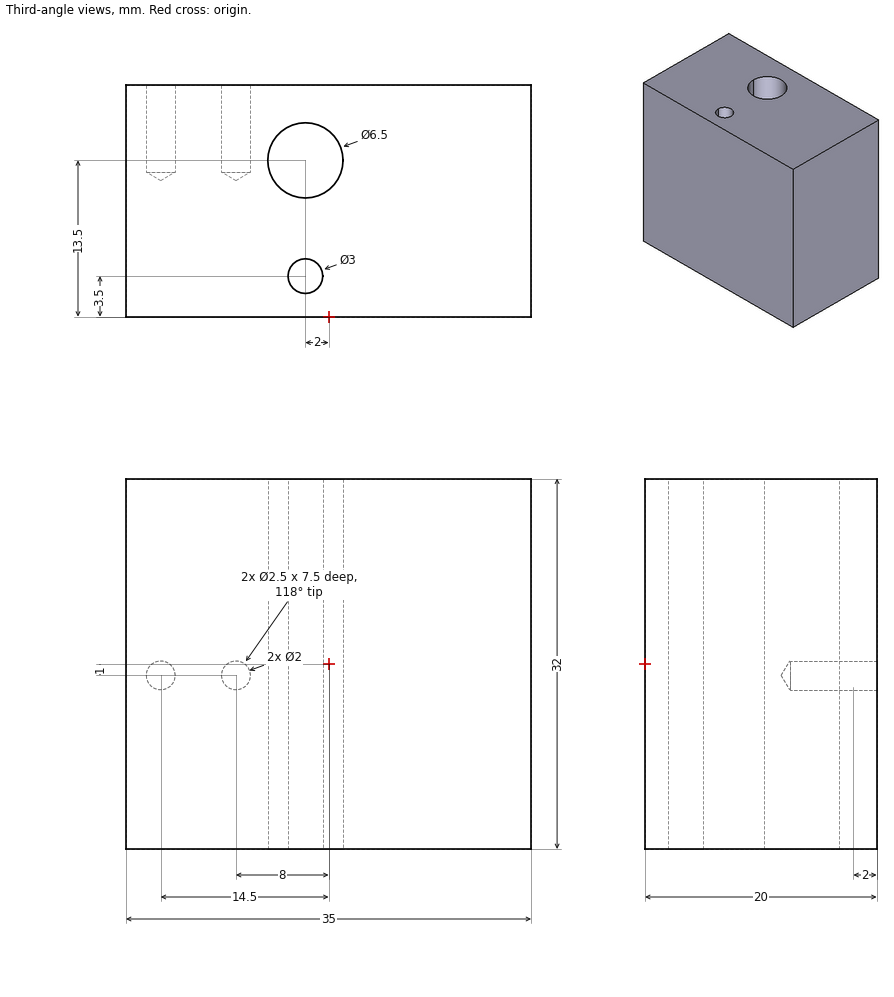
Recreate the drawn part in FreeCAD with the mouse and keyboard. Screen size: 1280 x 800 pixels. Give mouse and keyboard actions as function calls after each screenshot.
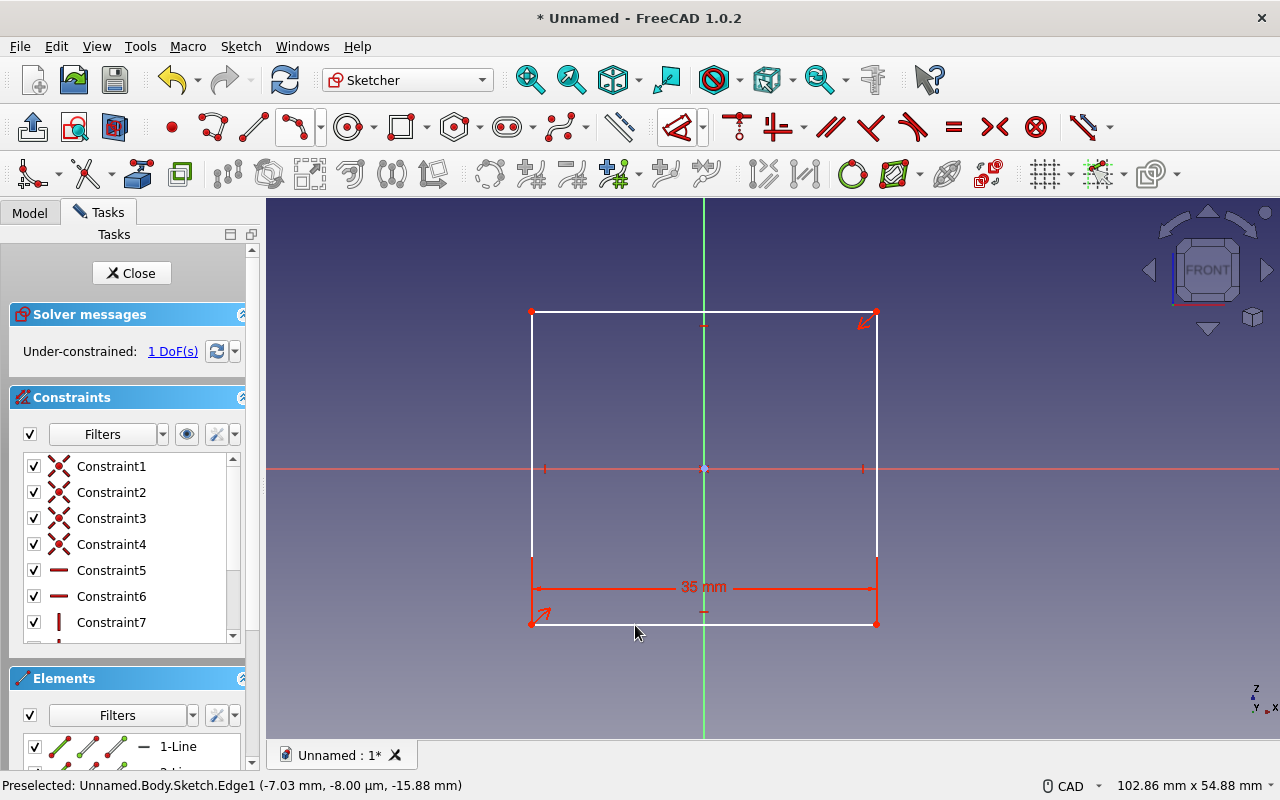
click(877, 531)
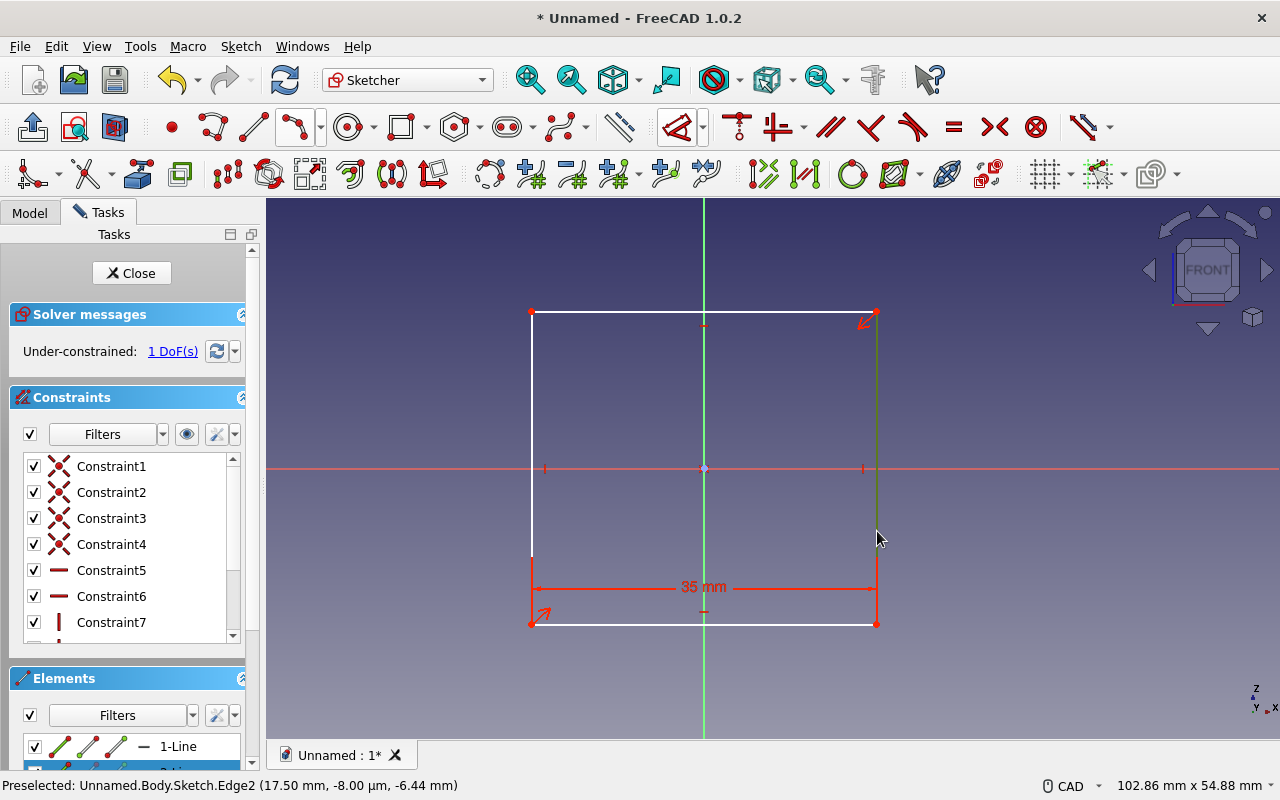
key(i)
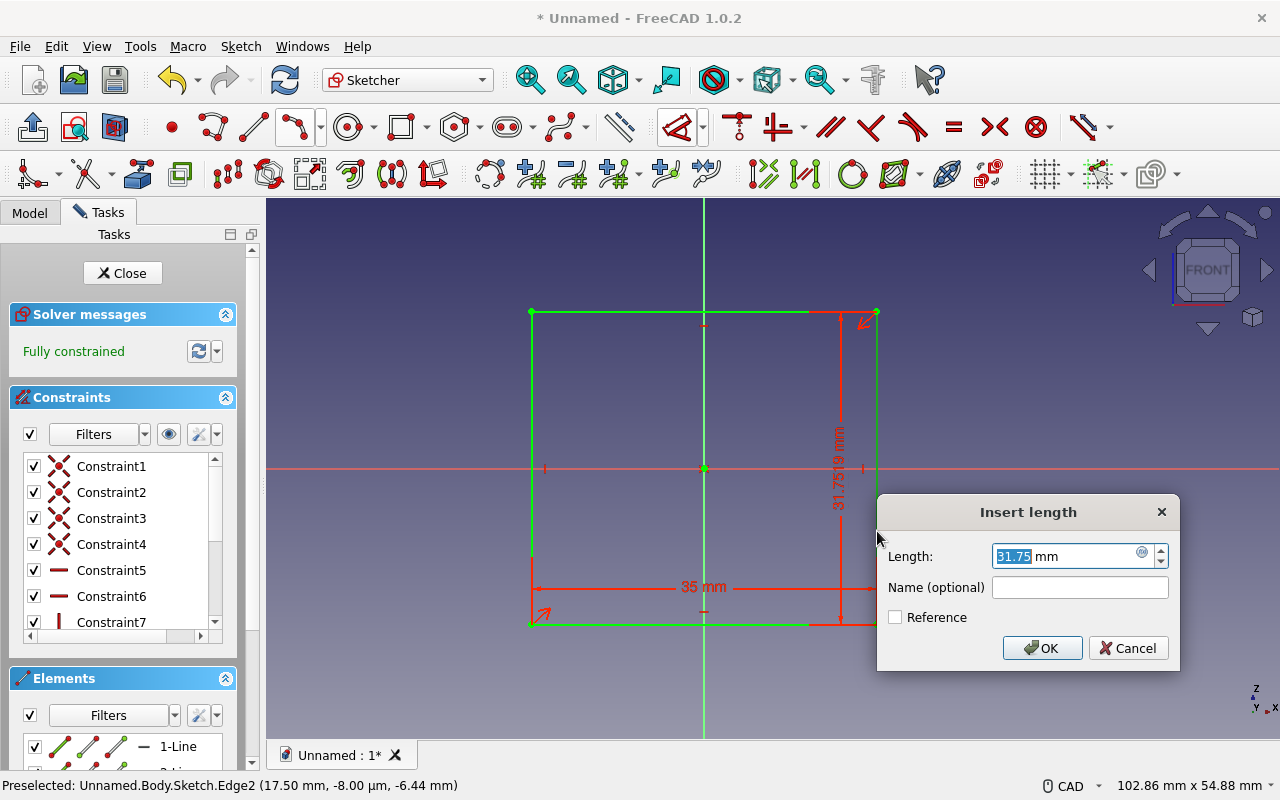
text(32)
key(Return)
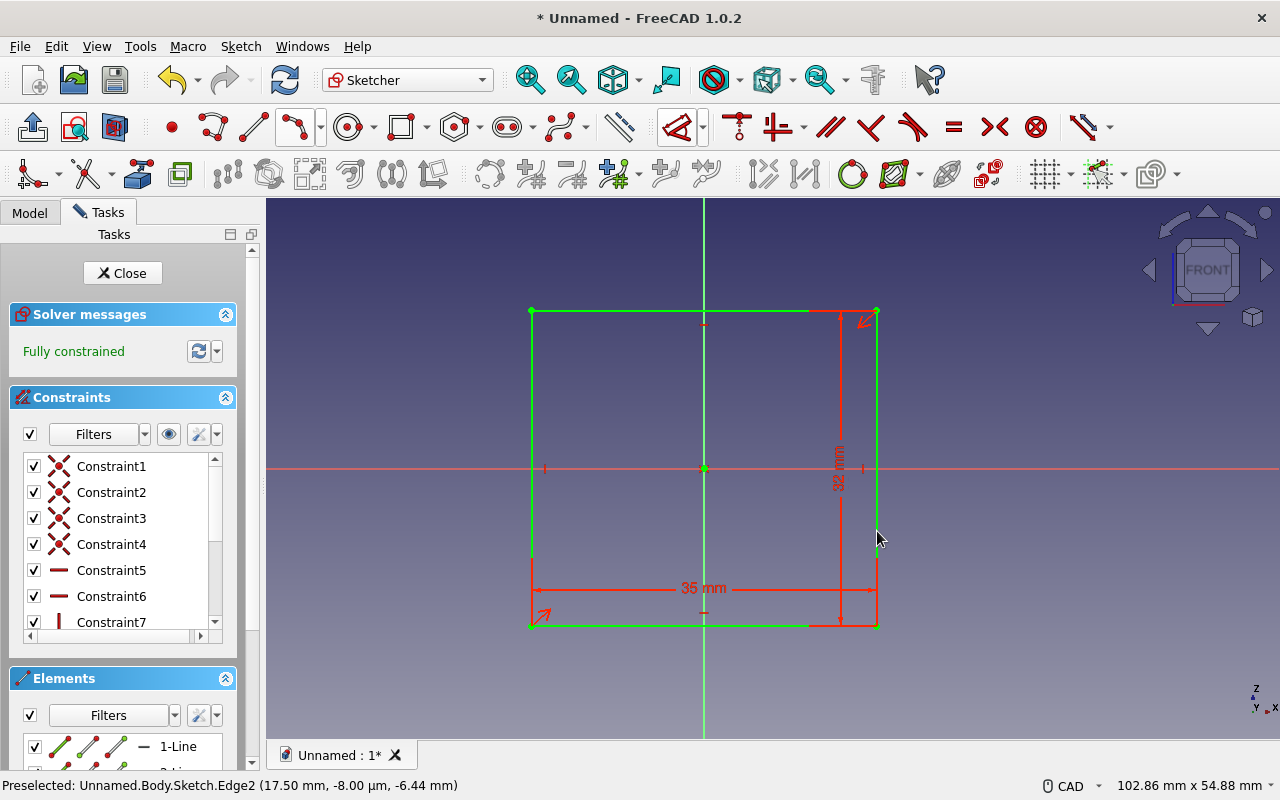
click(123, 273)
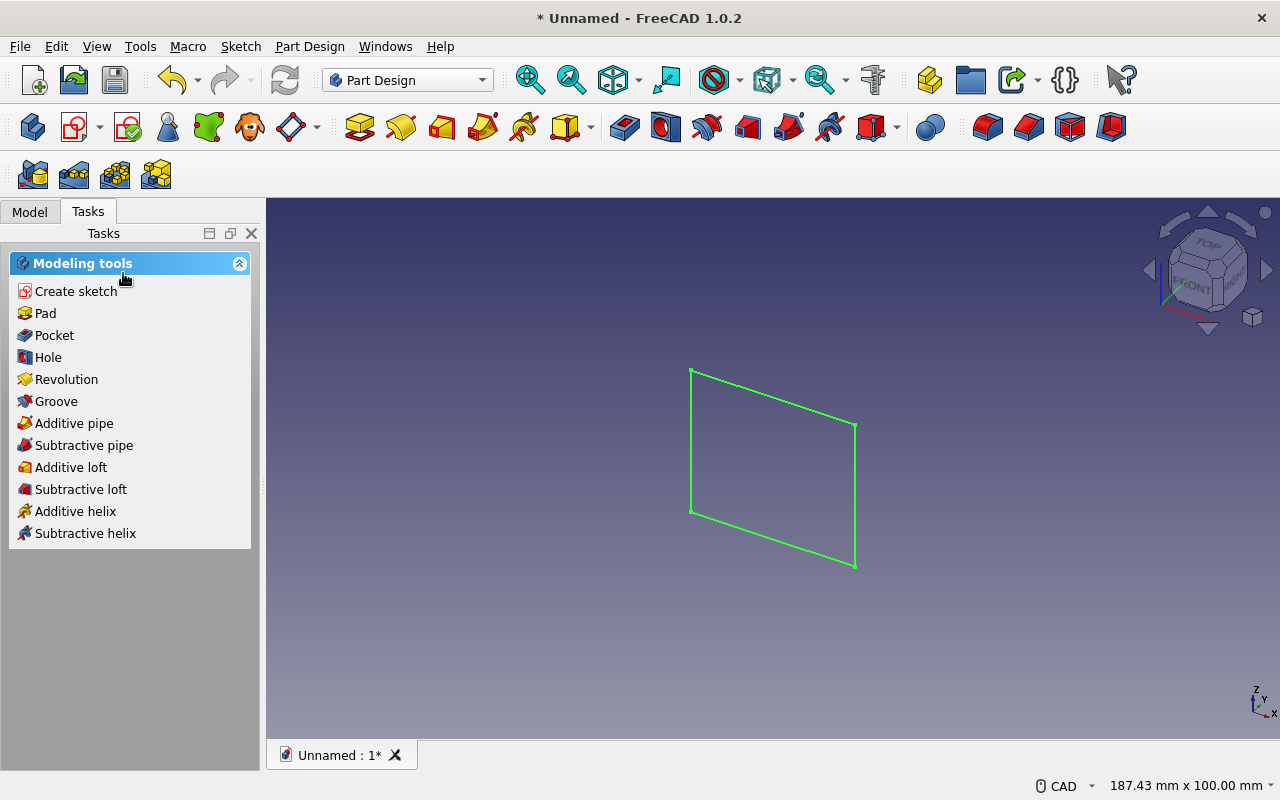
click(360, 128)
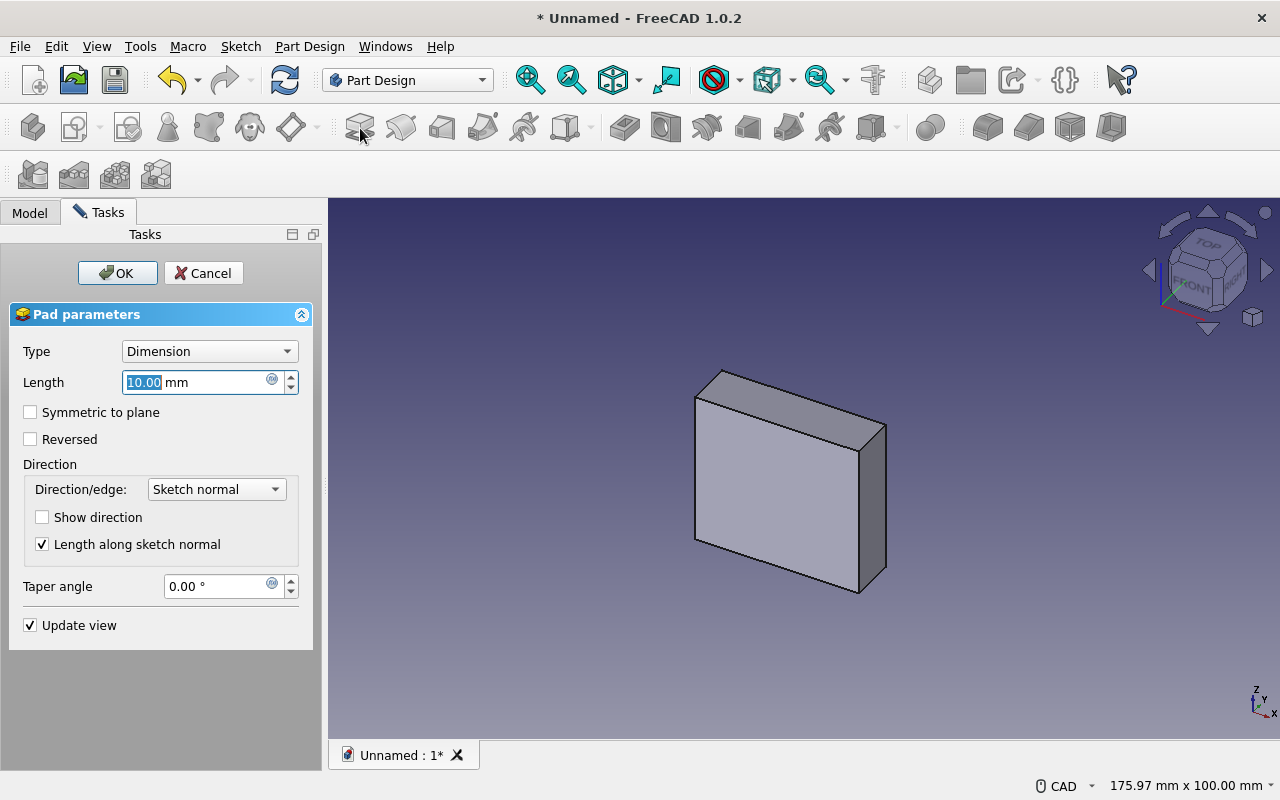
text(20)
key(Tab)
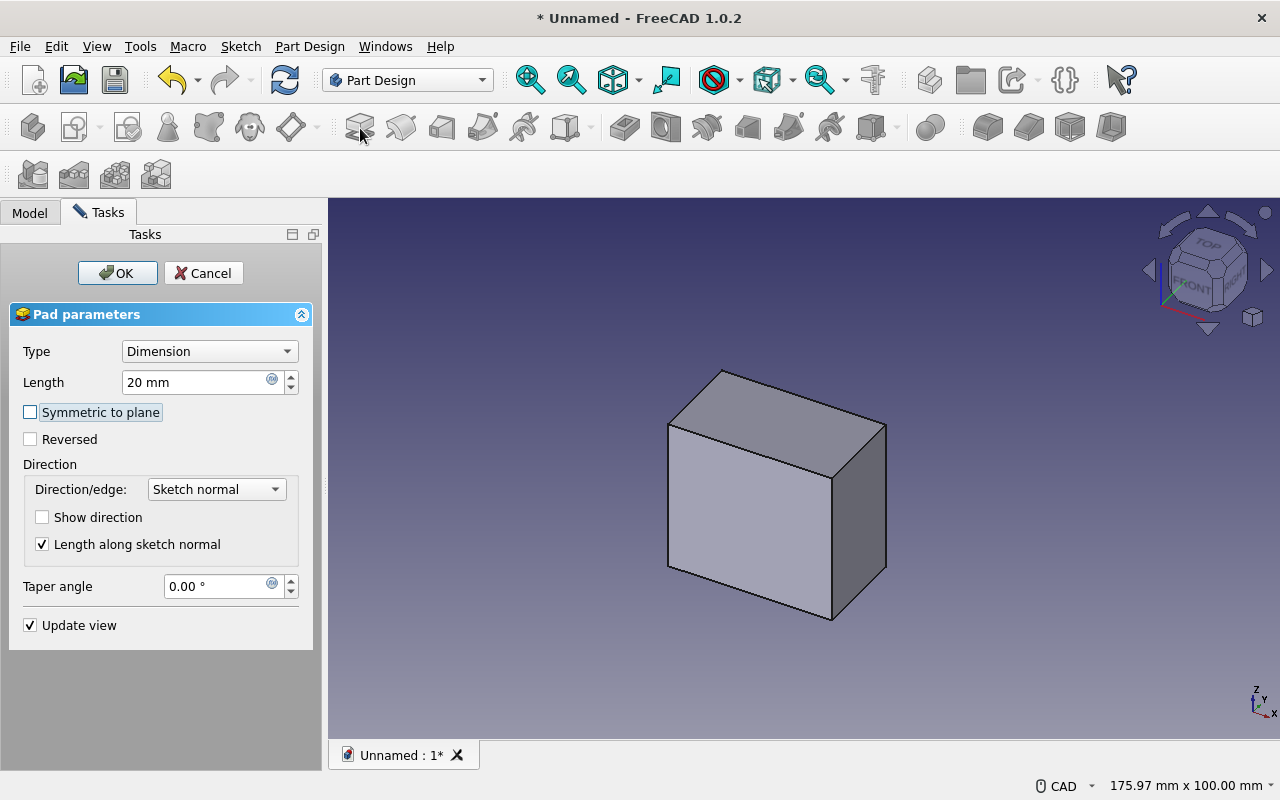
click(31, 439)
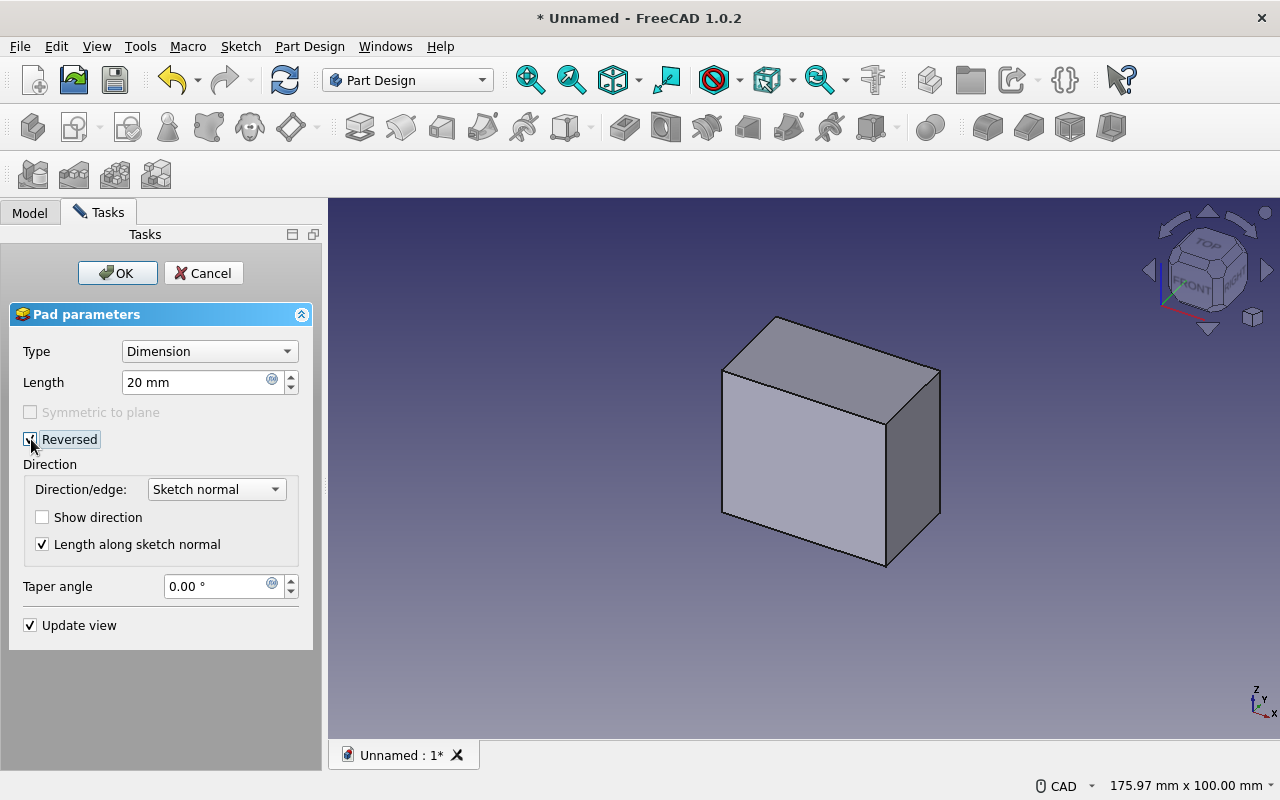
click(118, 273)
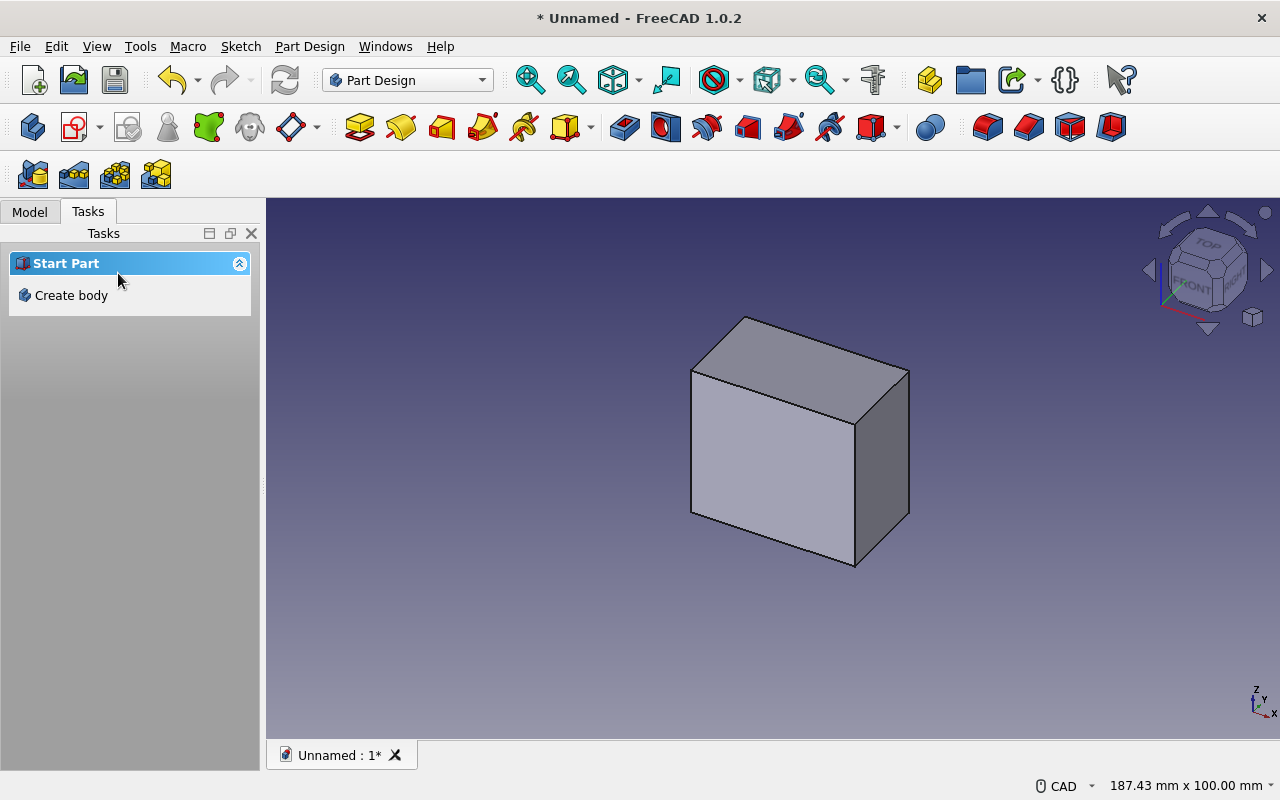
click(823, 377)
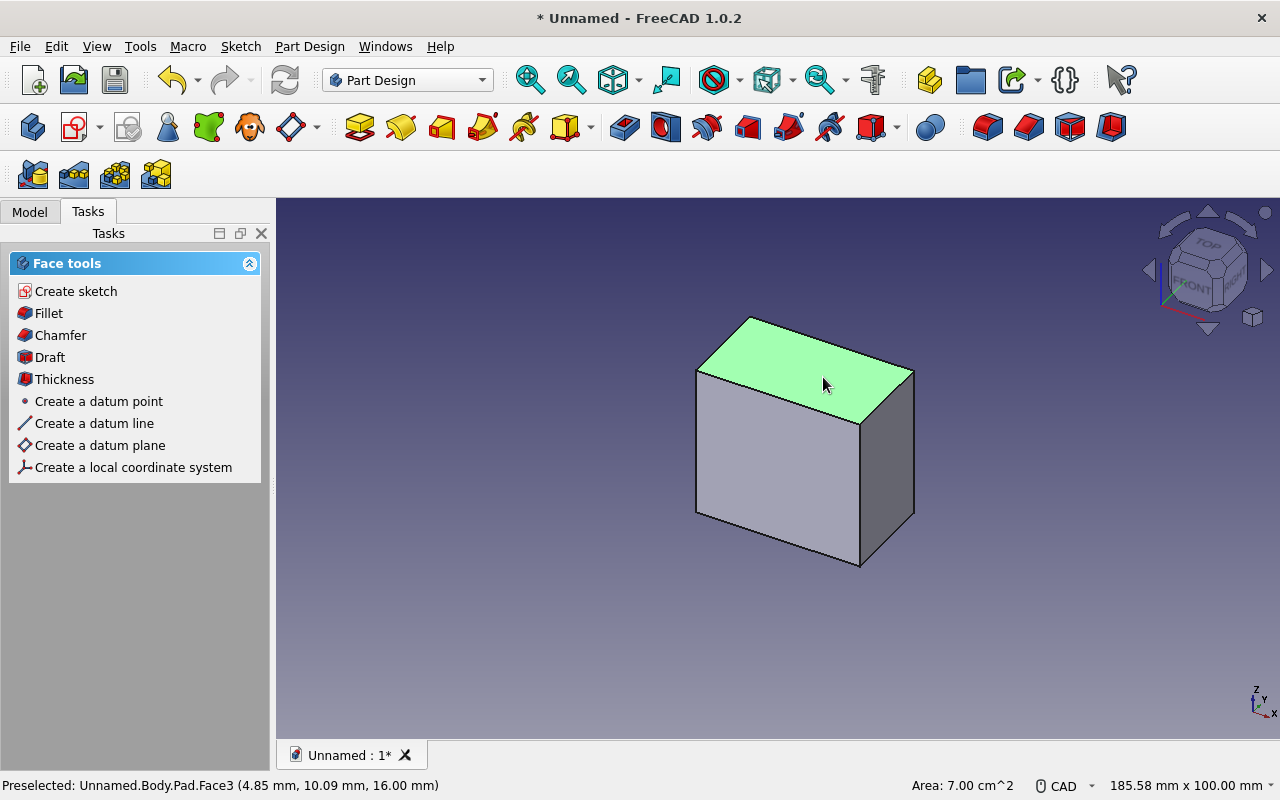
click(74, 128)